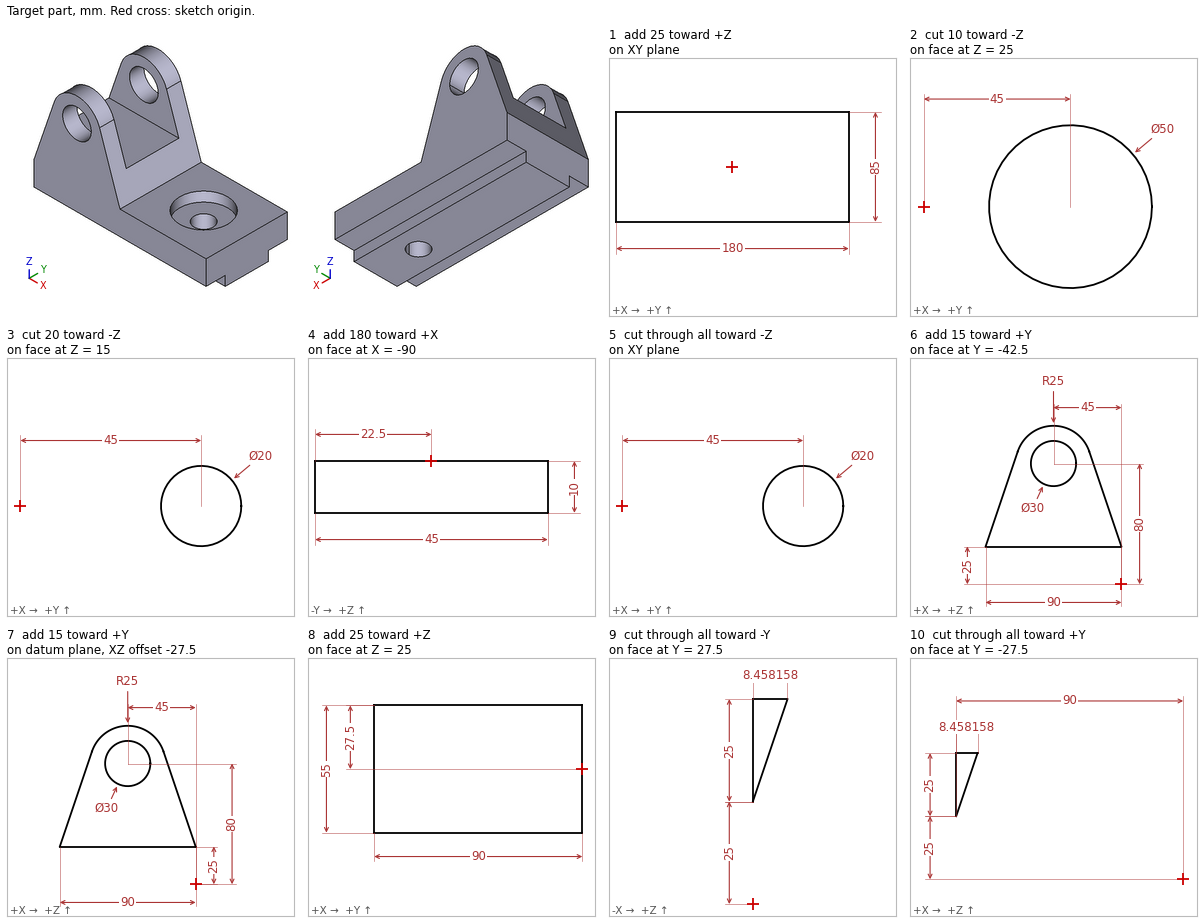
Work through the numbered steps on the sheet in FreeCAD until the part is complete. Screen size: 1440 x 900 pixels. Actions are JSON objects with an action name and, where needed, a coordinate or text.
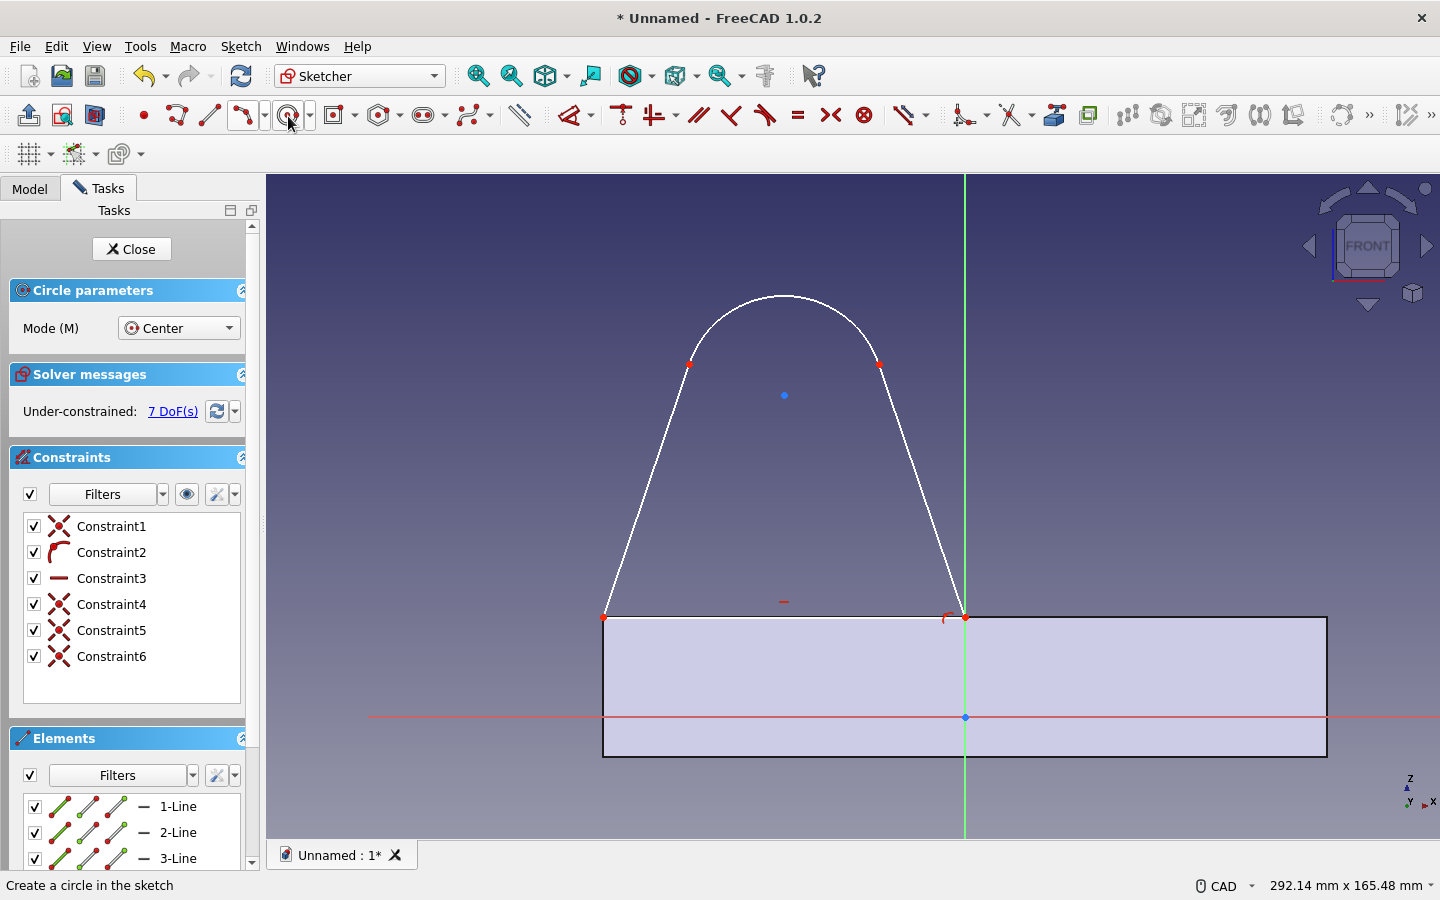
{"action": "left_click", "coordinate": [784, 396]}
{"action": "mouse_move", "coordinate": [827, 353]}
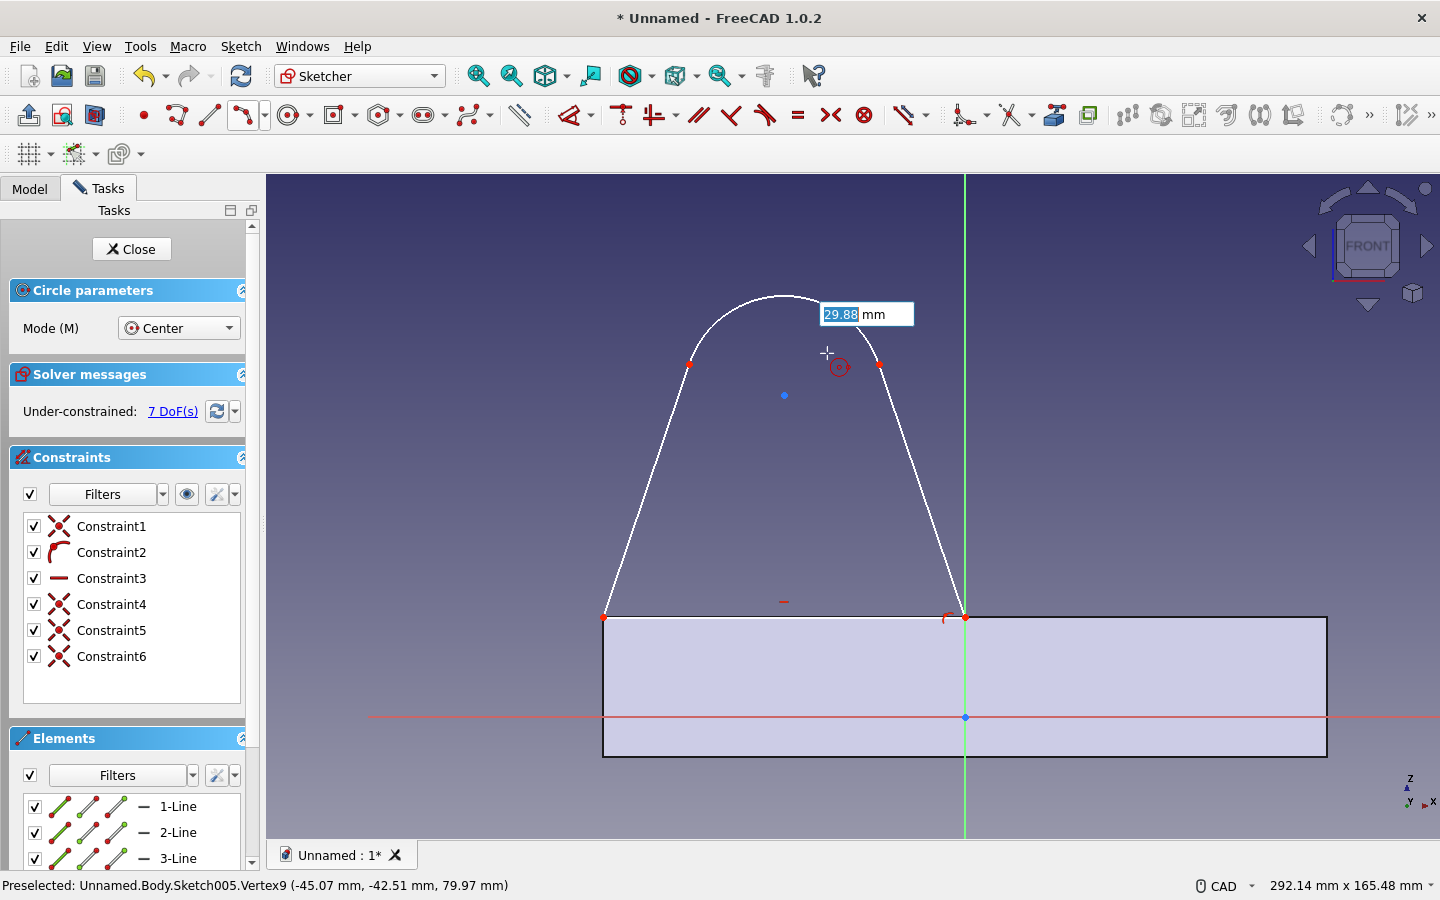
{"action": "type", "text": "30"}
{"action": "key", "text": "Return"}
{"action": "key", "text": "Escape"}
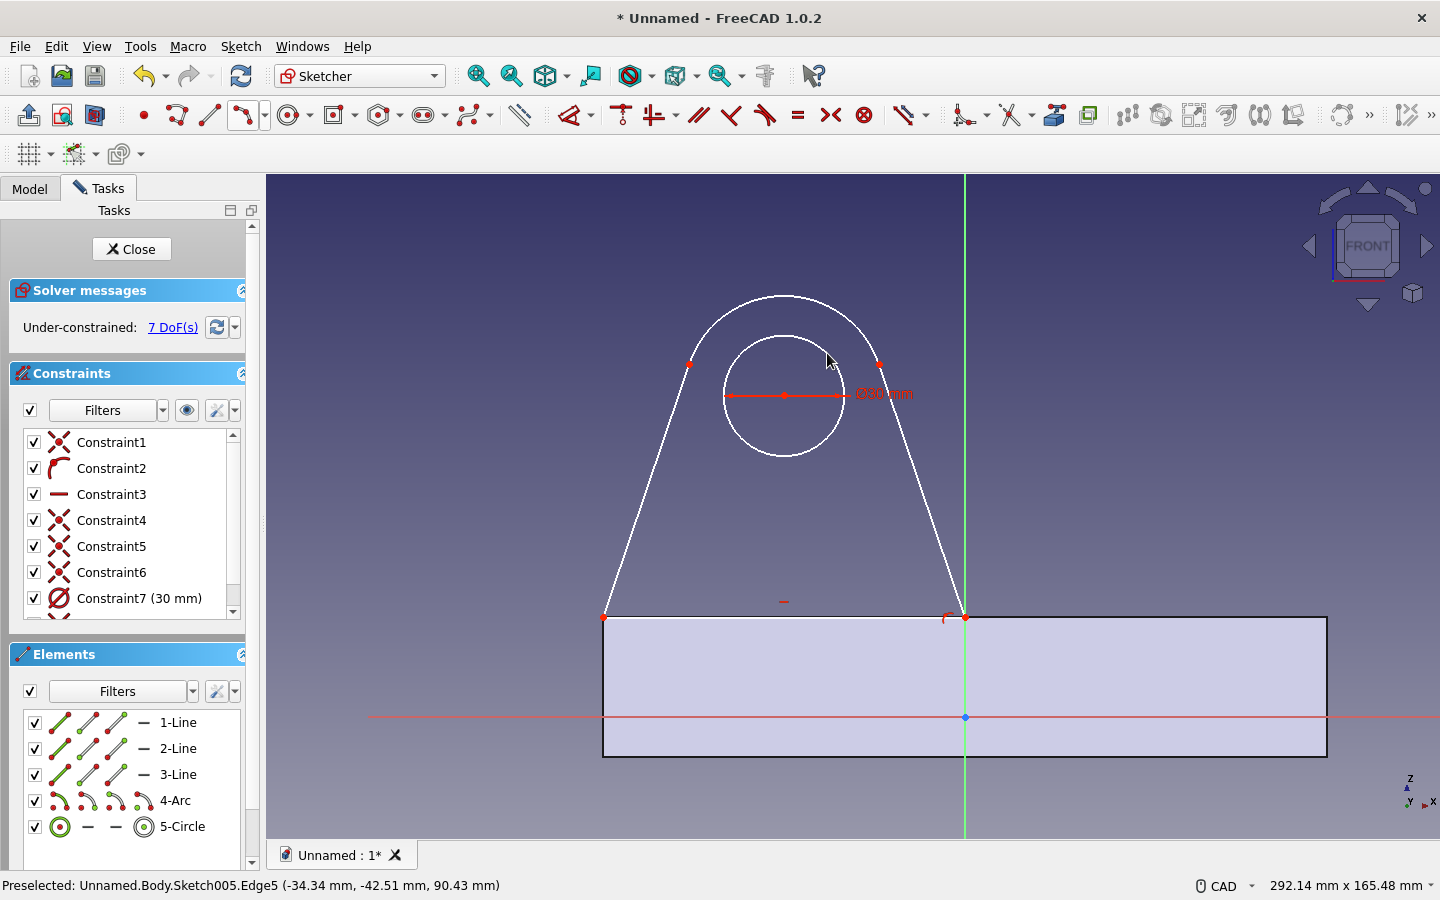
{"action": "left_click", "coordinate": [663, 441]}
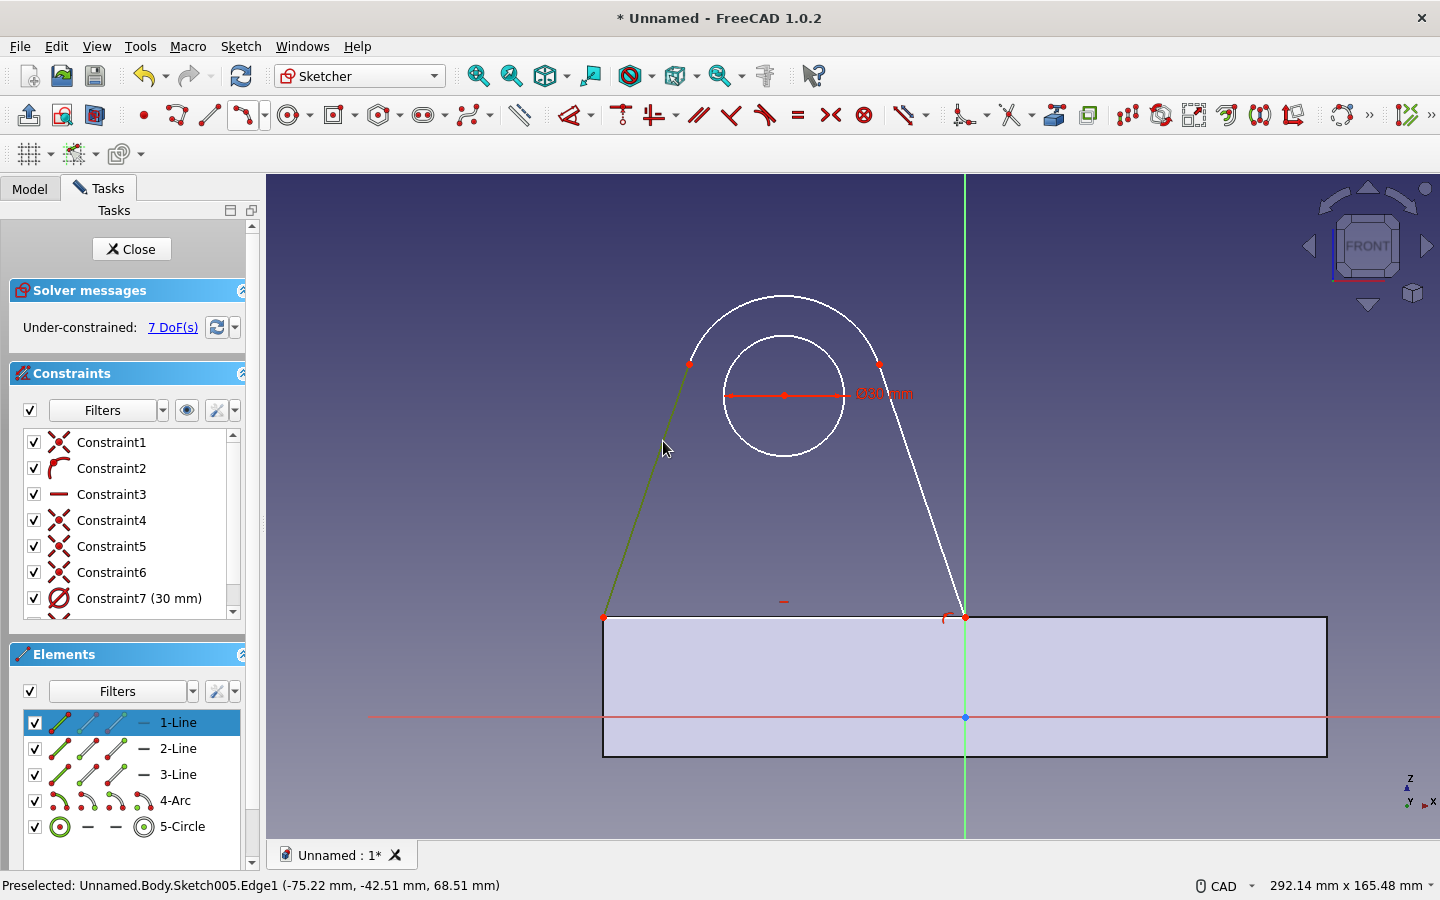
{"action": "left_click", "coordinate": [832, 308]}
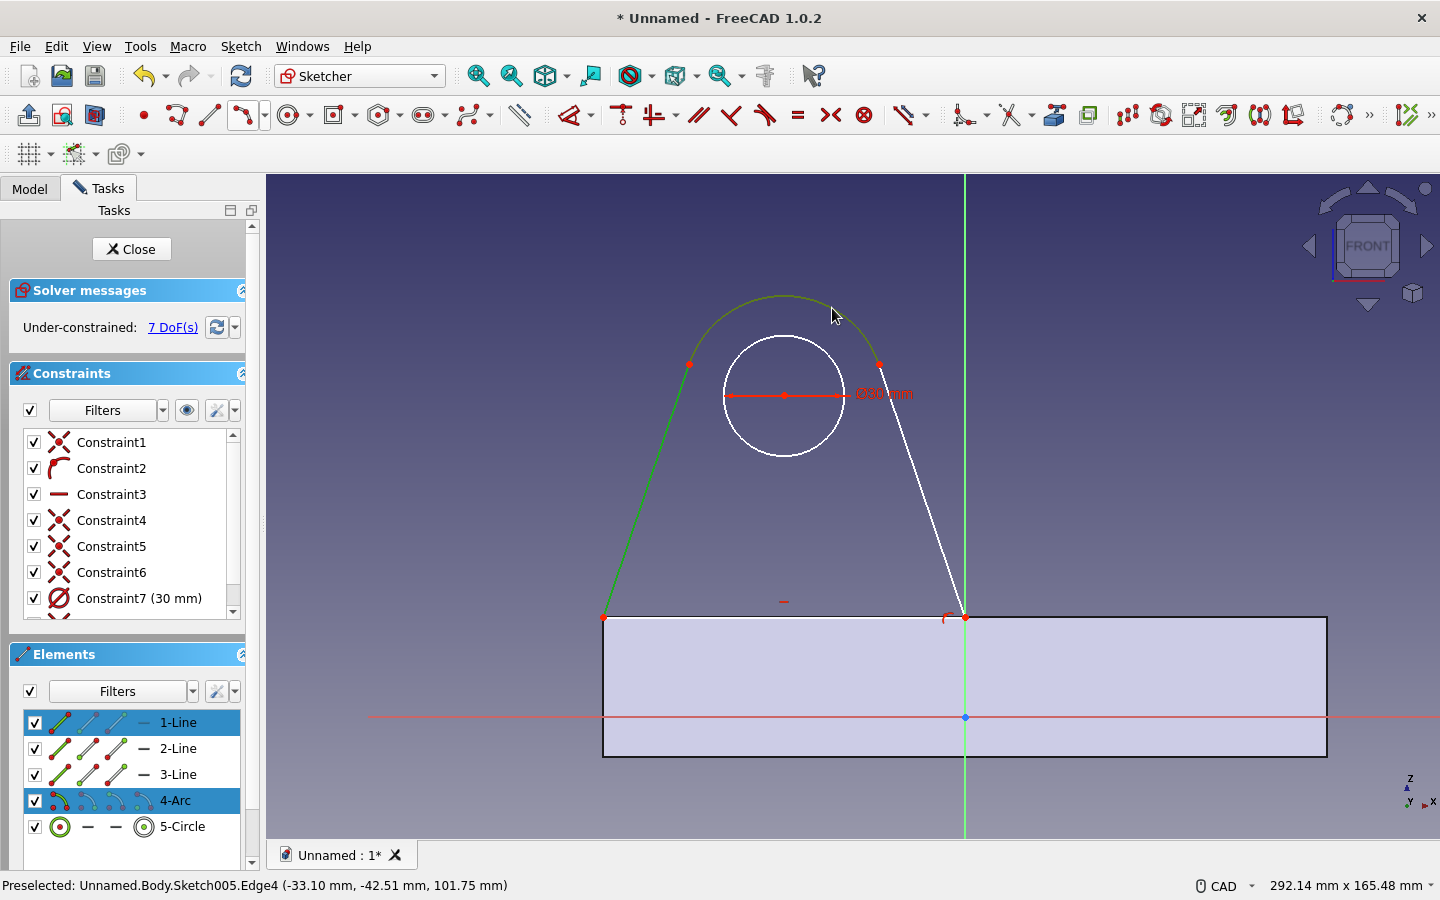
{"action": "left_click", "coordinate": [765, 116]}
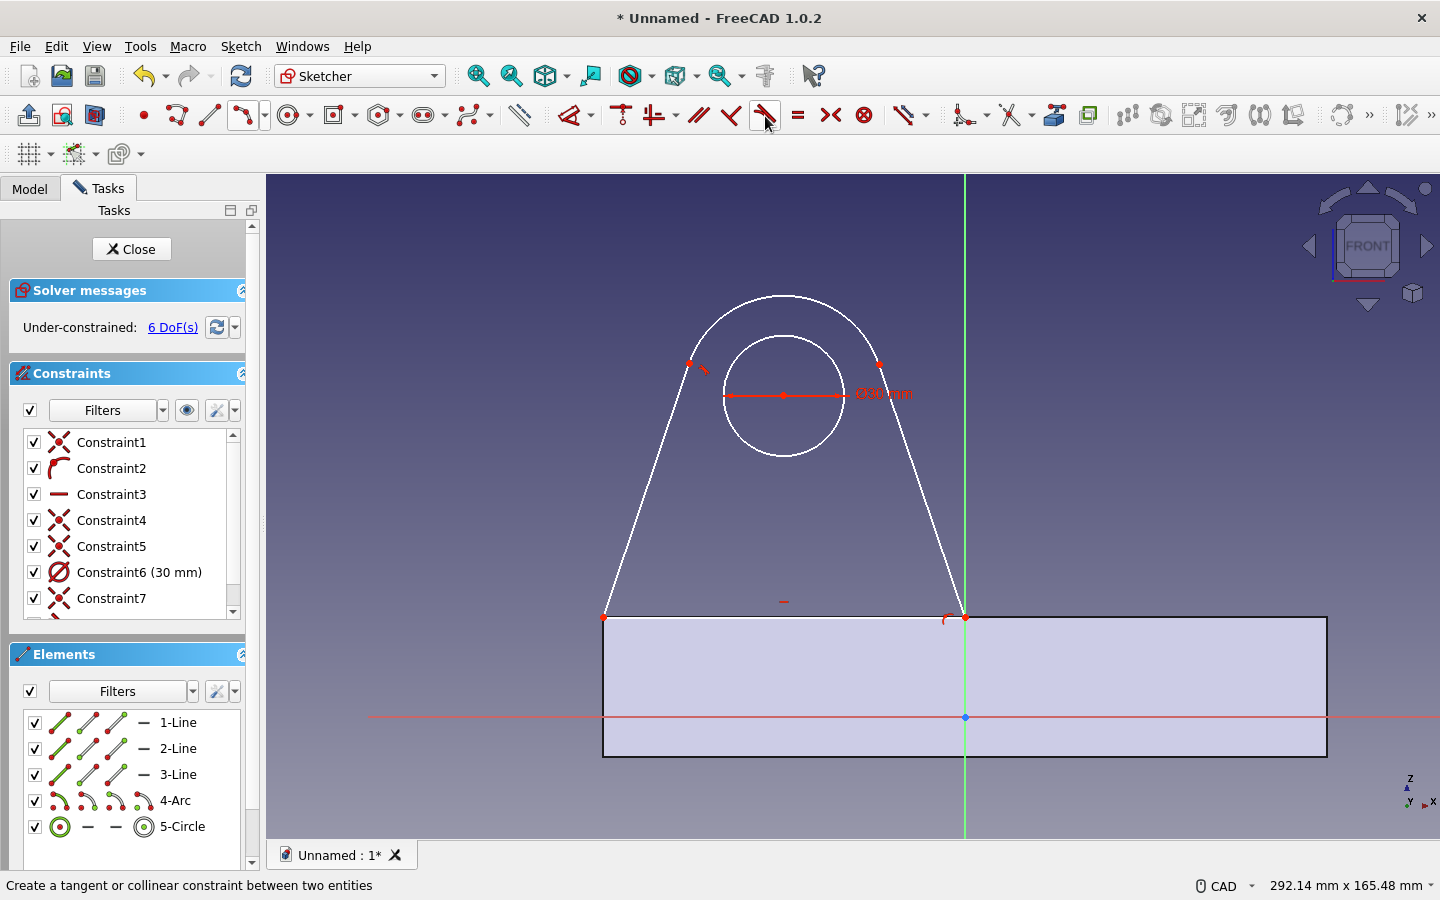
{"action": "left_click", "coordinate": [939, 542]}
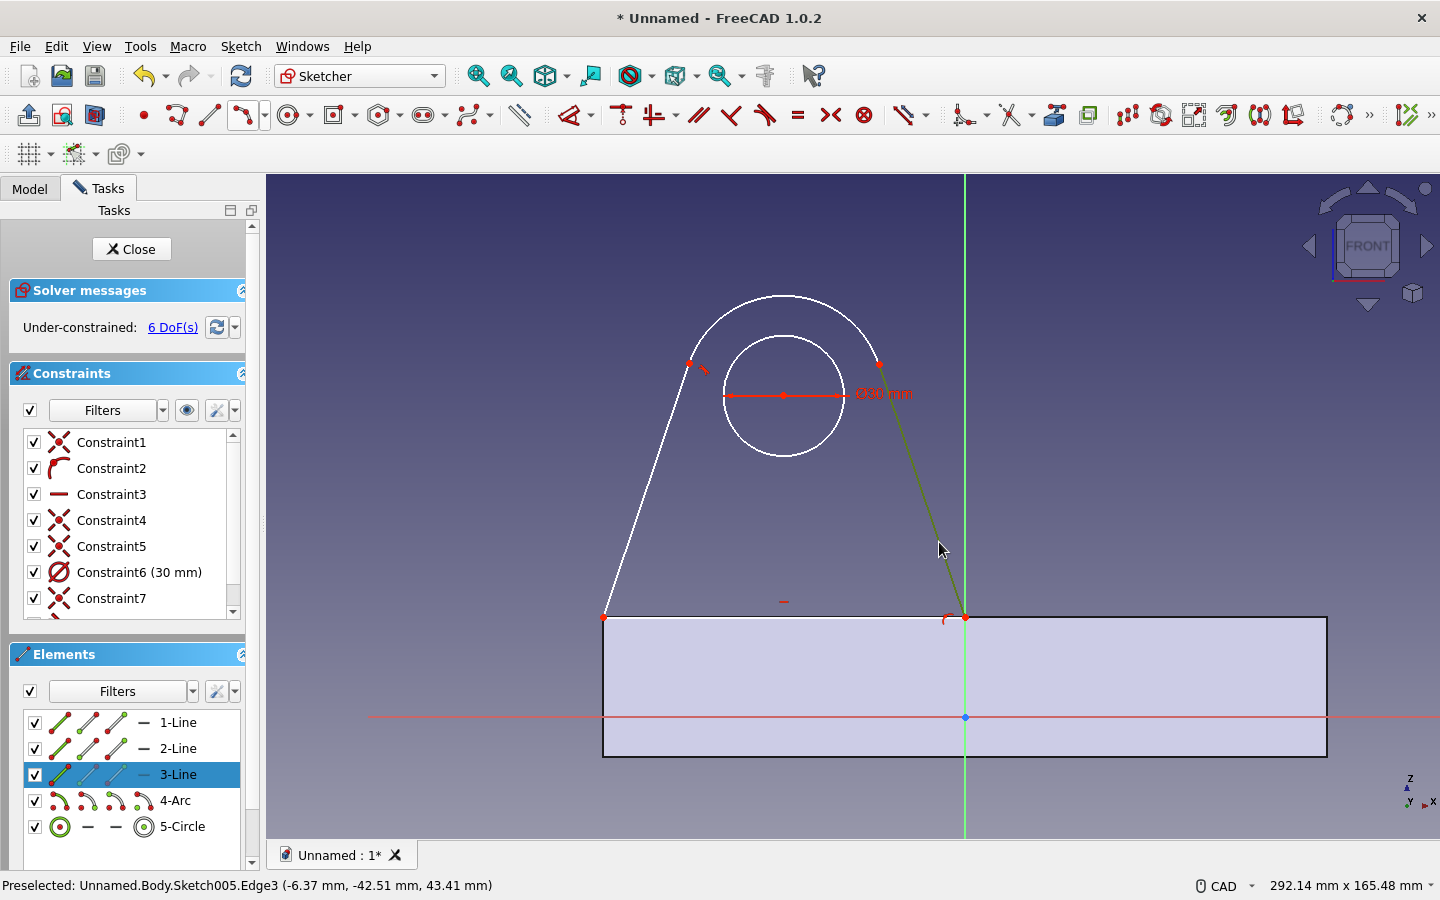
{"action": "left_click", "coordinate": [832, 308]}